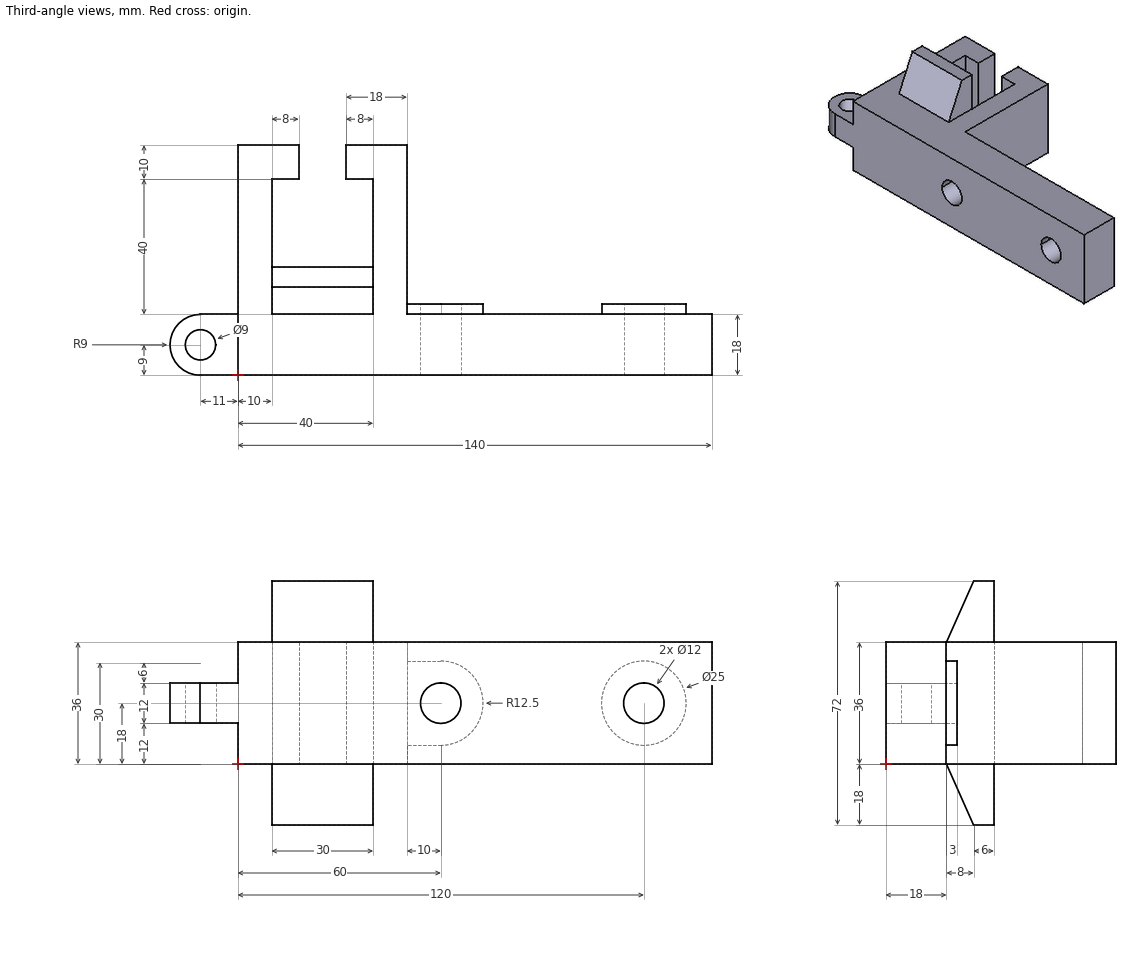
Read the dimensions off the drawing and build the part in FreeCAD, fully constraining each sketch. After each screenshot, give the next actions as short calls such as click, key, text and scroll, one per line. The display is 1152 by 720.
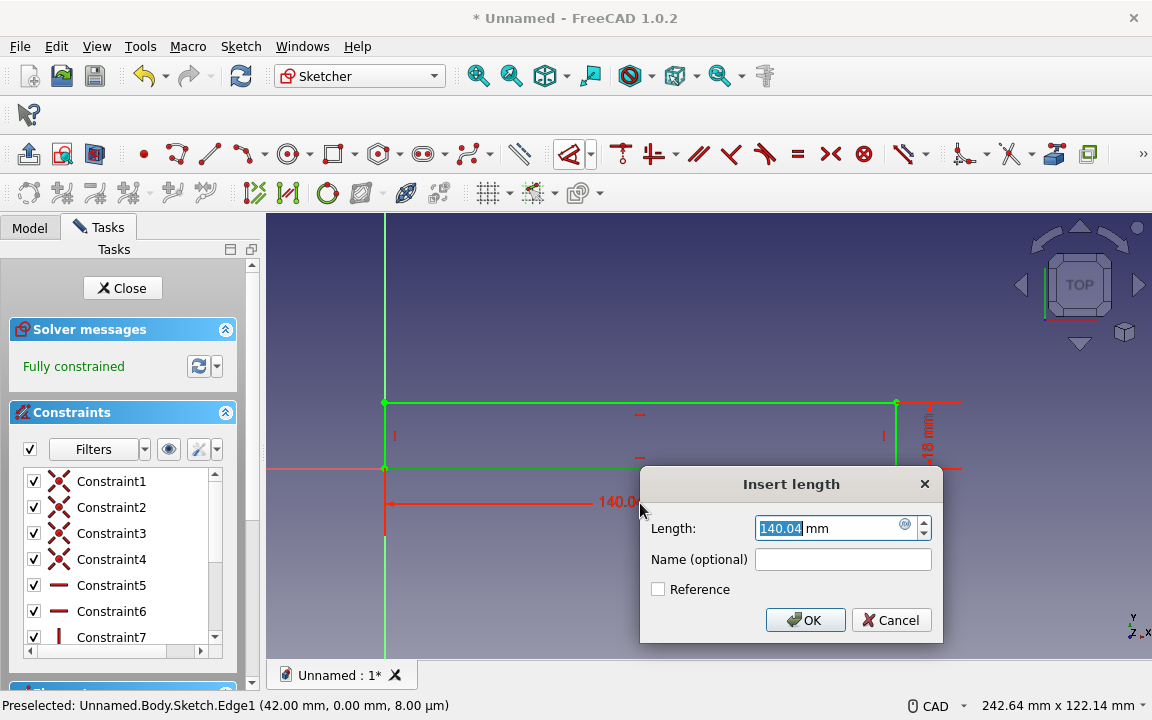
text(140)
key(Return)
key(Escape)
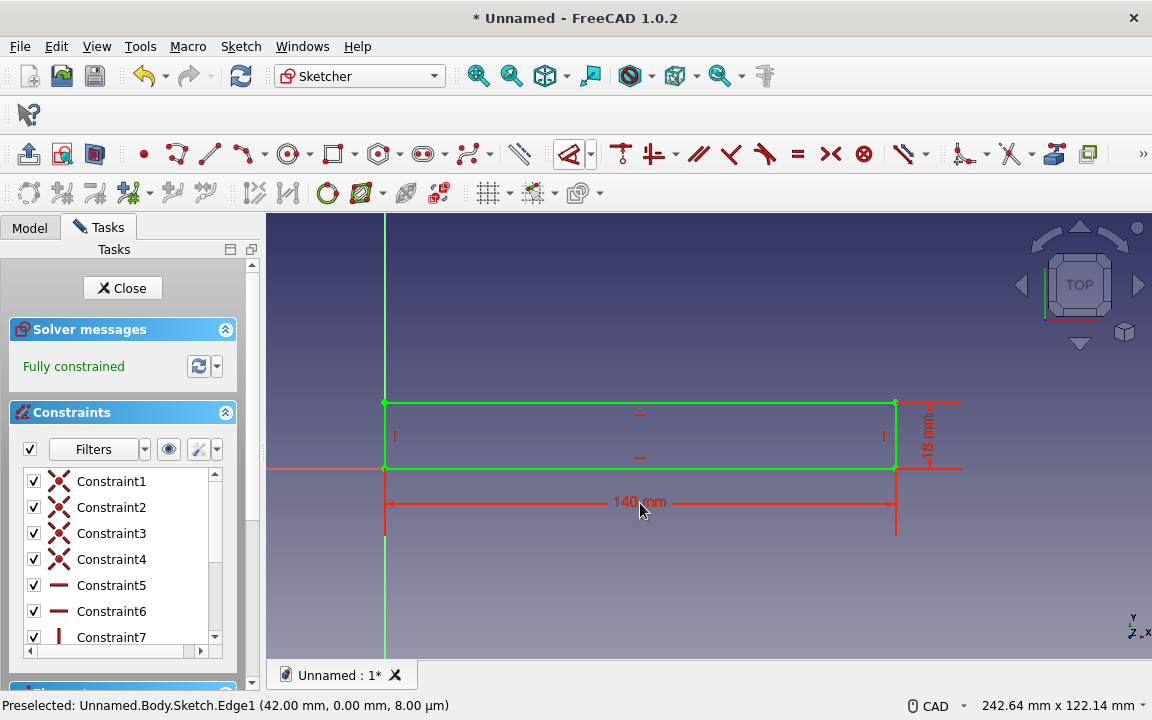
click(123, 288)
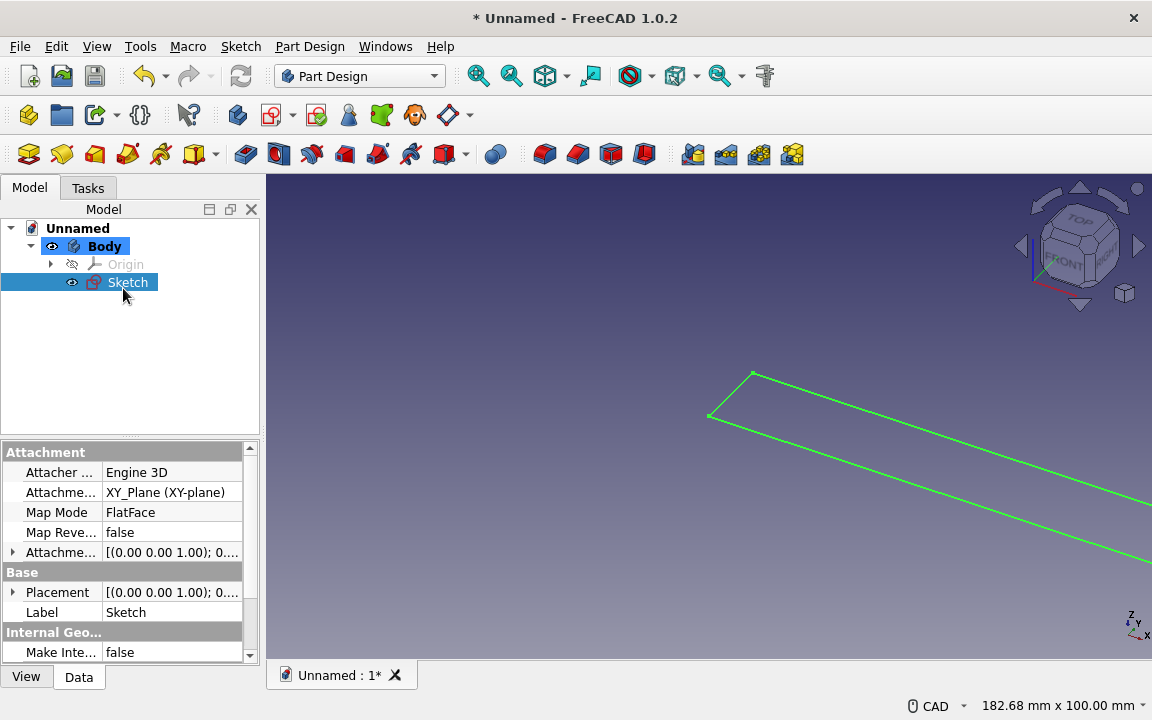
click(29, 154)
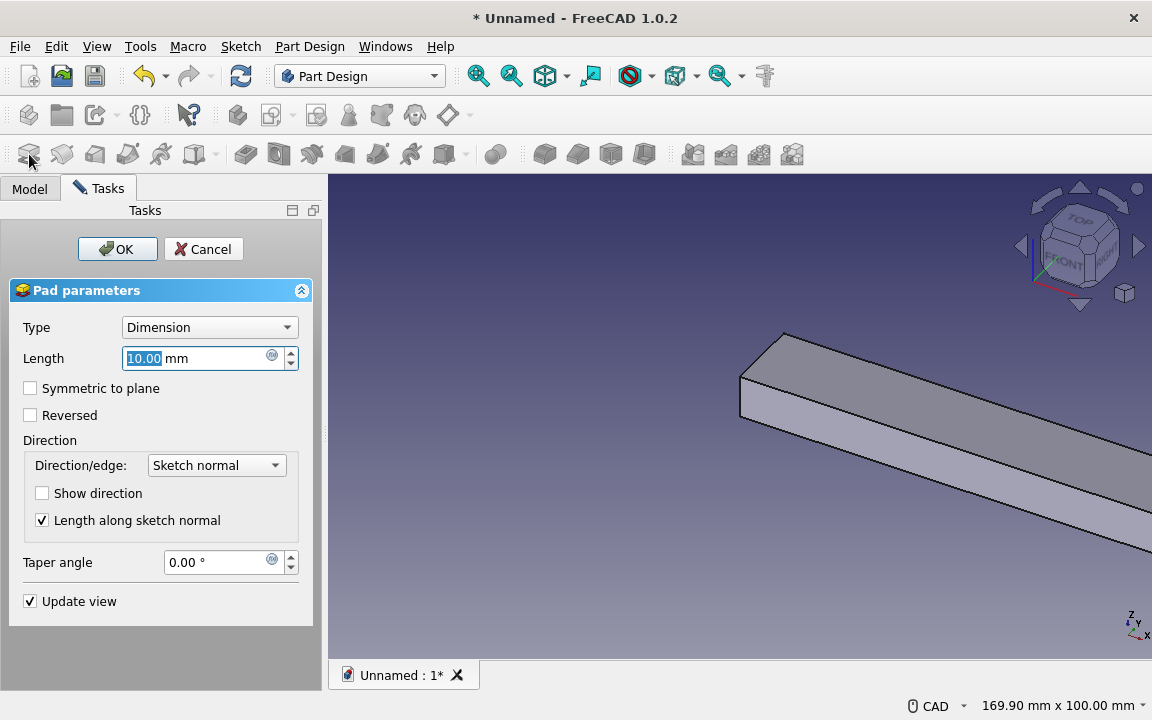
text(36)
key(Tab)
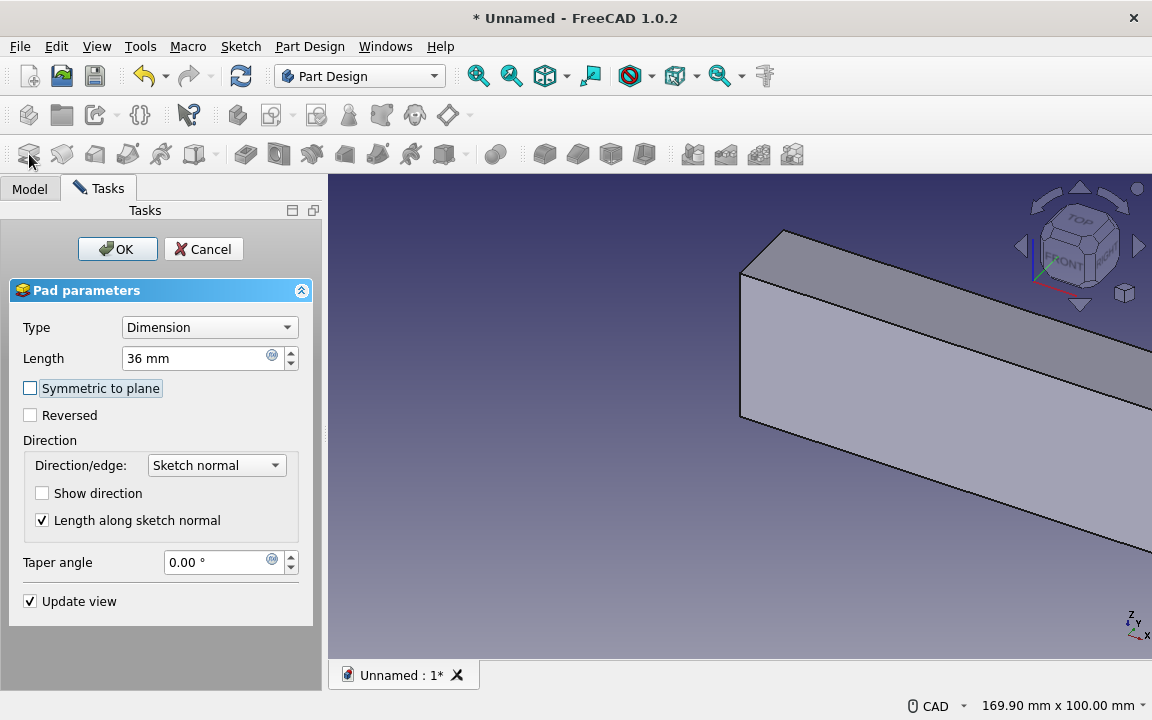
click(118, 249)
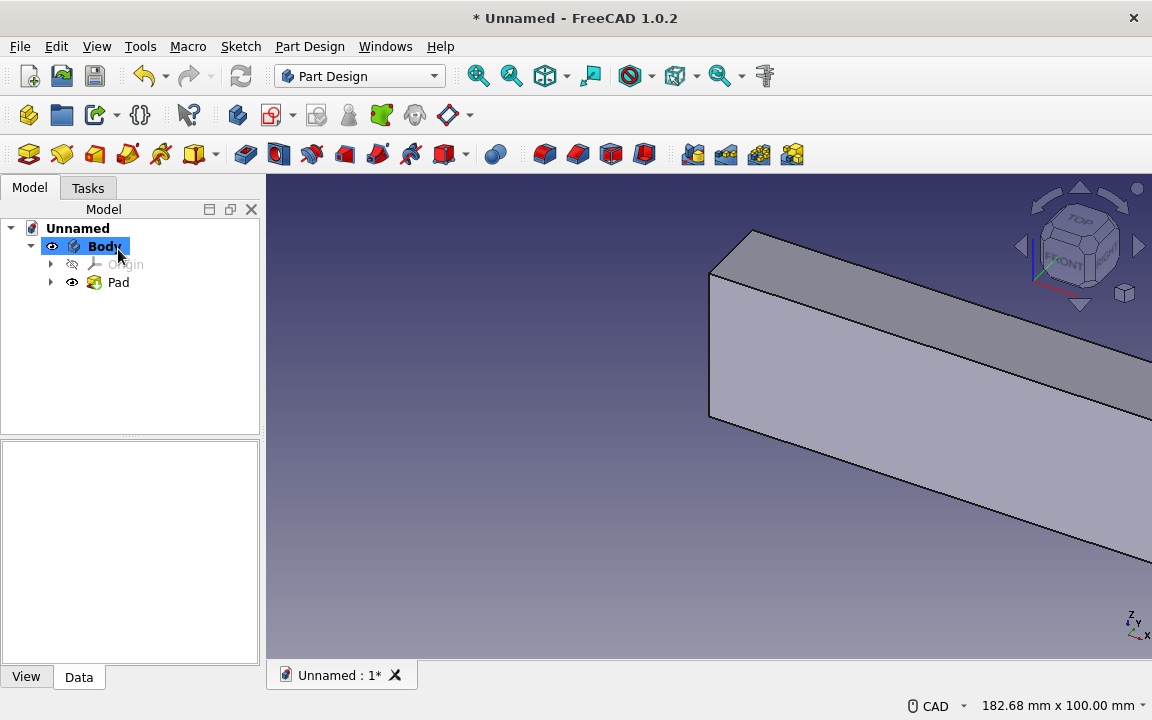
key(v)
key(f)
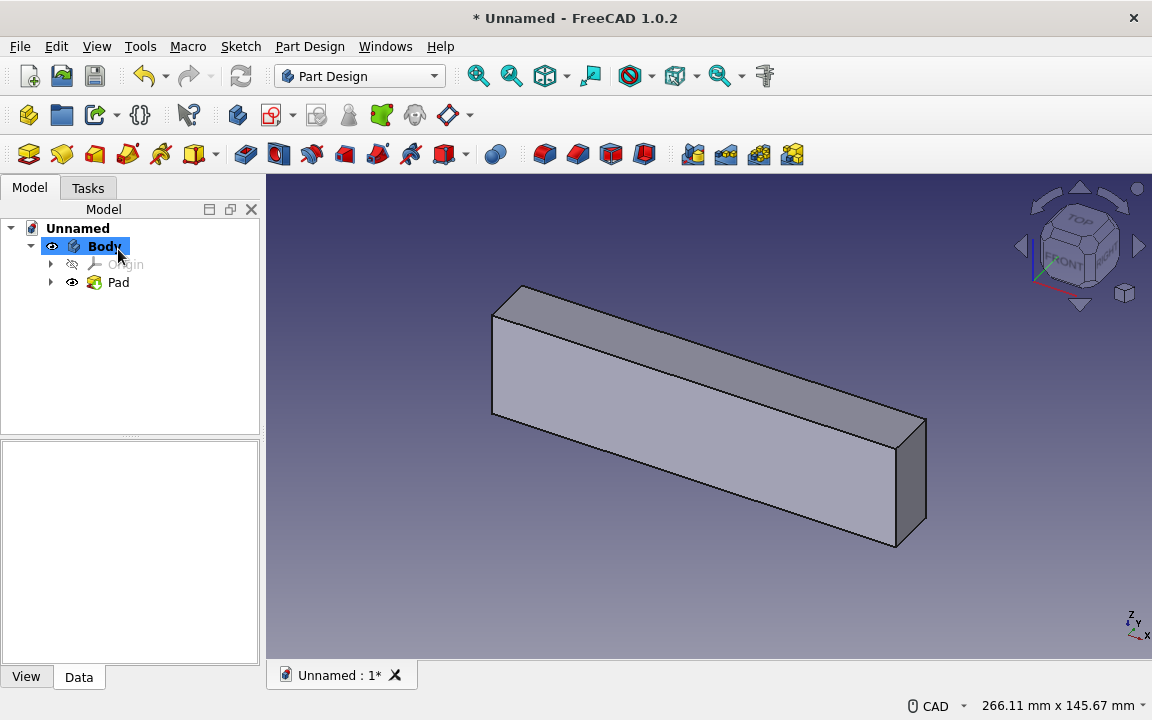
click(882, 424)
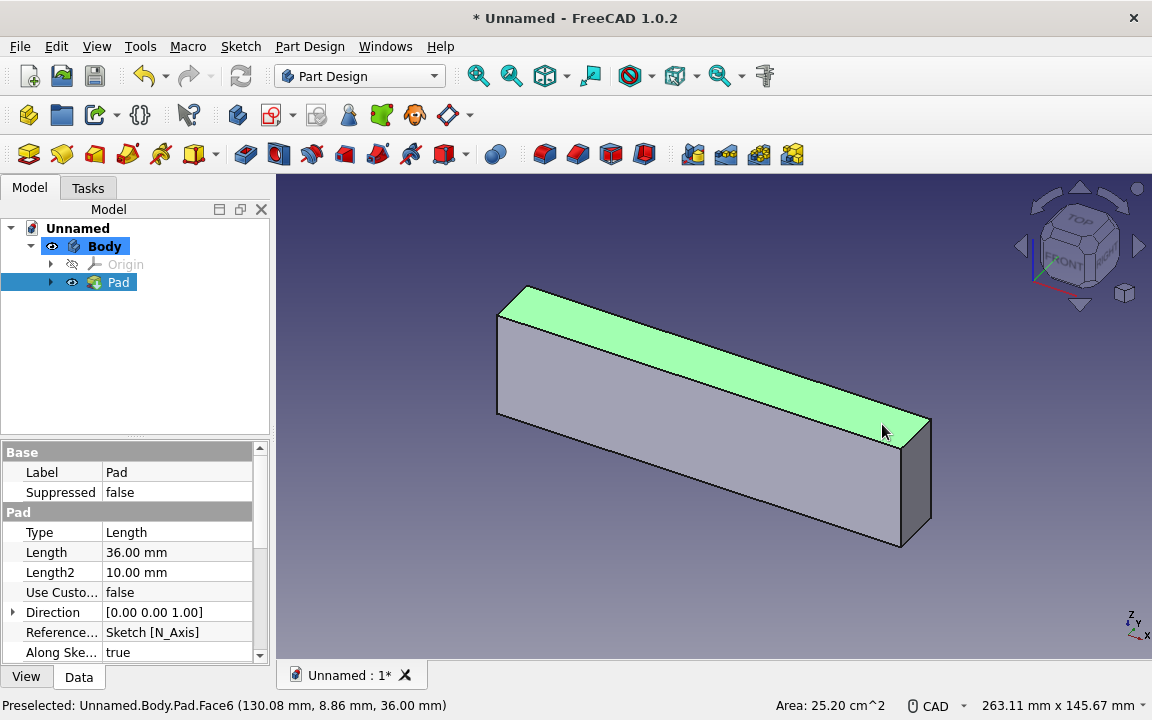
click(270, 116)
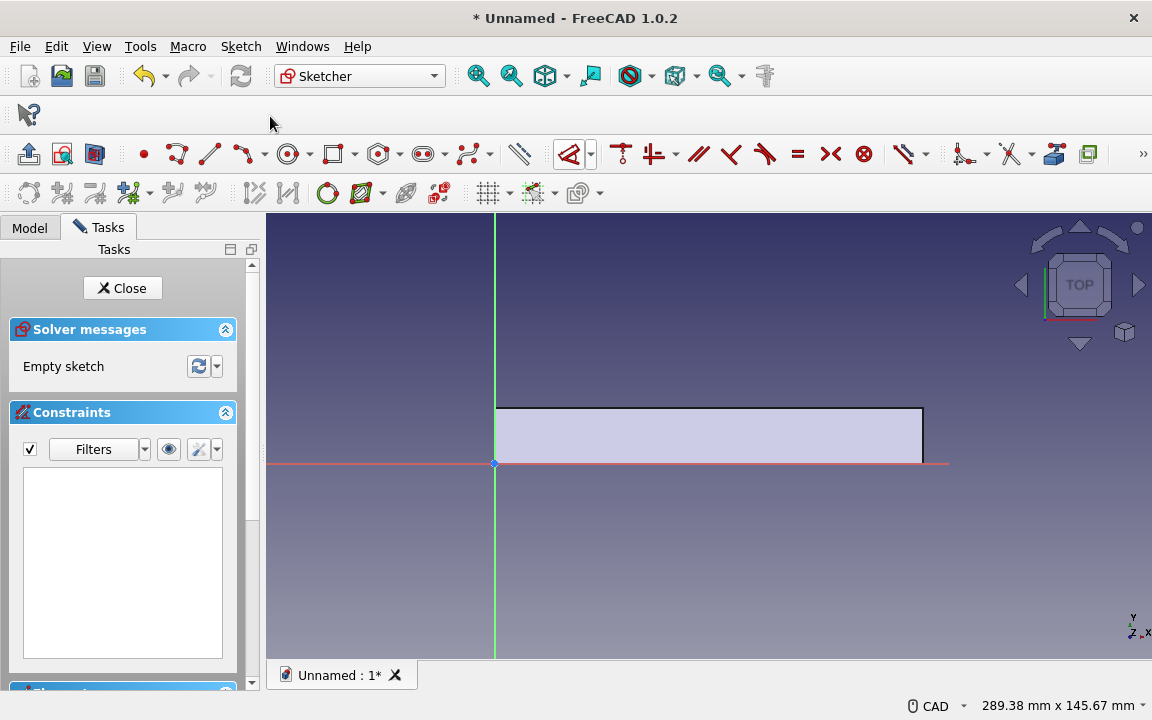
scroll(987, 631, down, 1)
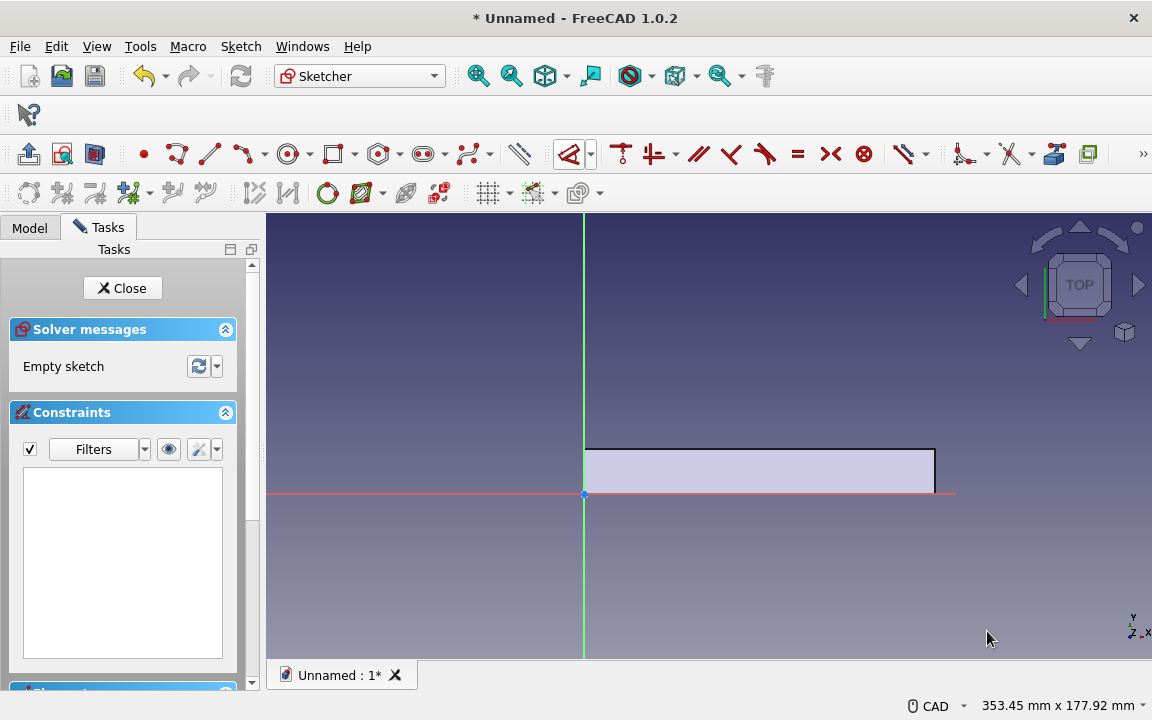
scroll(538, 354, up, 2)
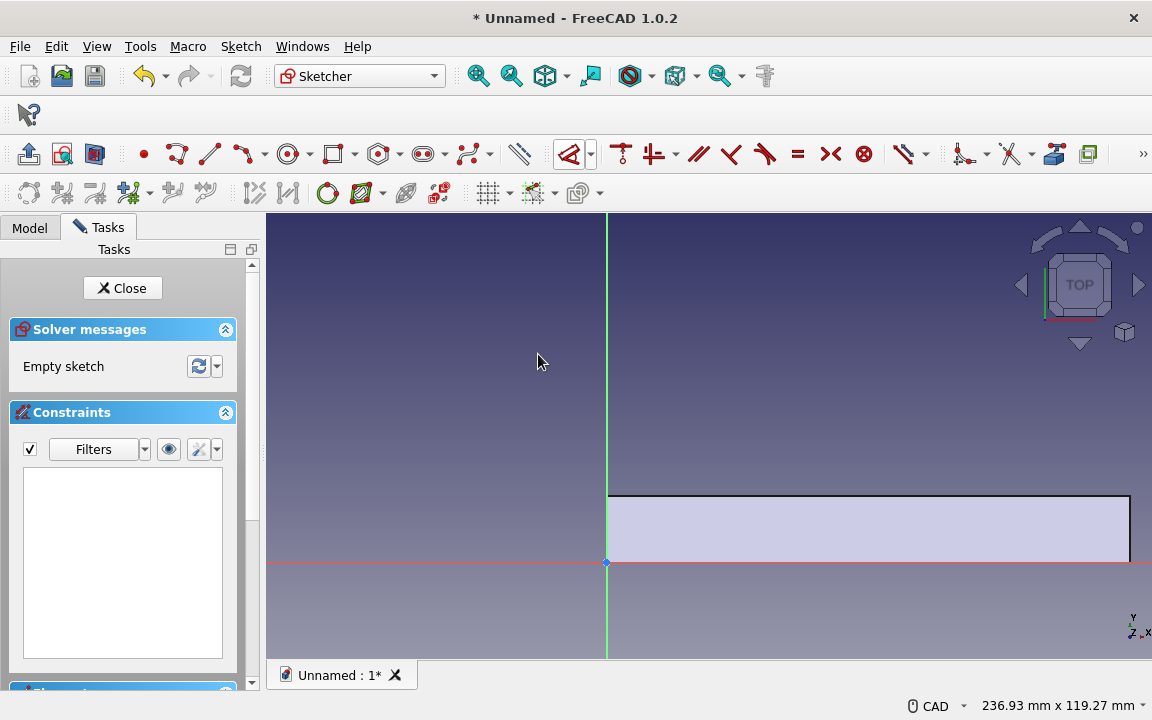
key(g)
key(m)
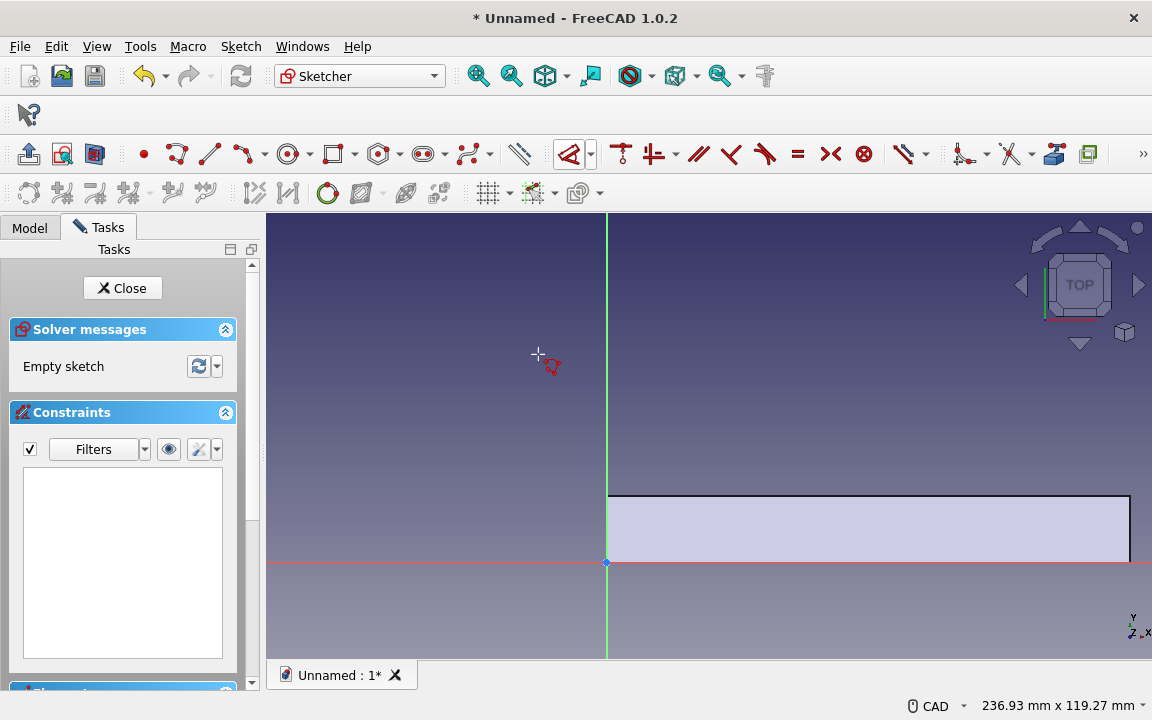
click(607, 496)
click(644, 496)
click(644, 346)
click(674, 346)
click(674, 309)
click(616, 309)
click(607, 497)
key(Escape)
key(Escape)